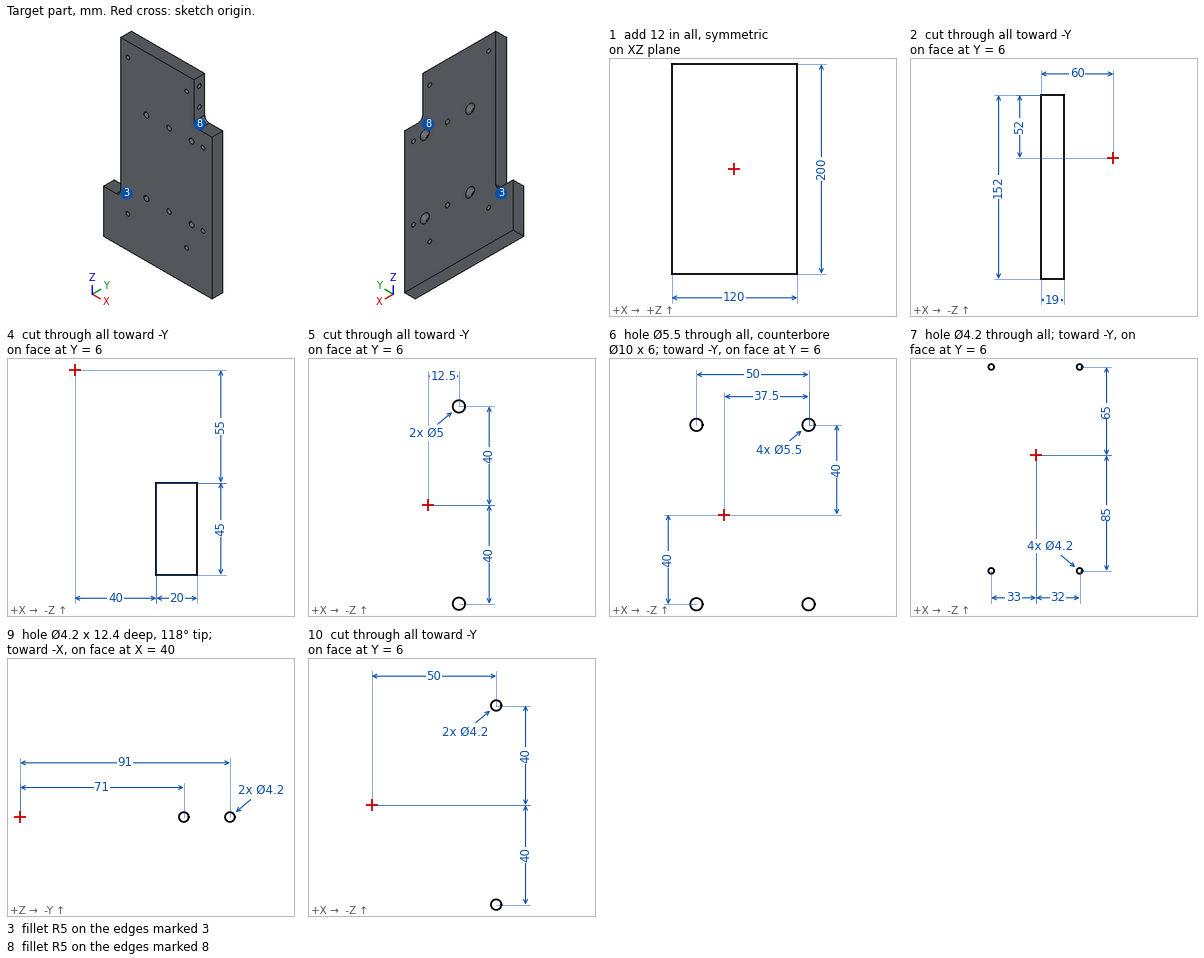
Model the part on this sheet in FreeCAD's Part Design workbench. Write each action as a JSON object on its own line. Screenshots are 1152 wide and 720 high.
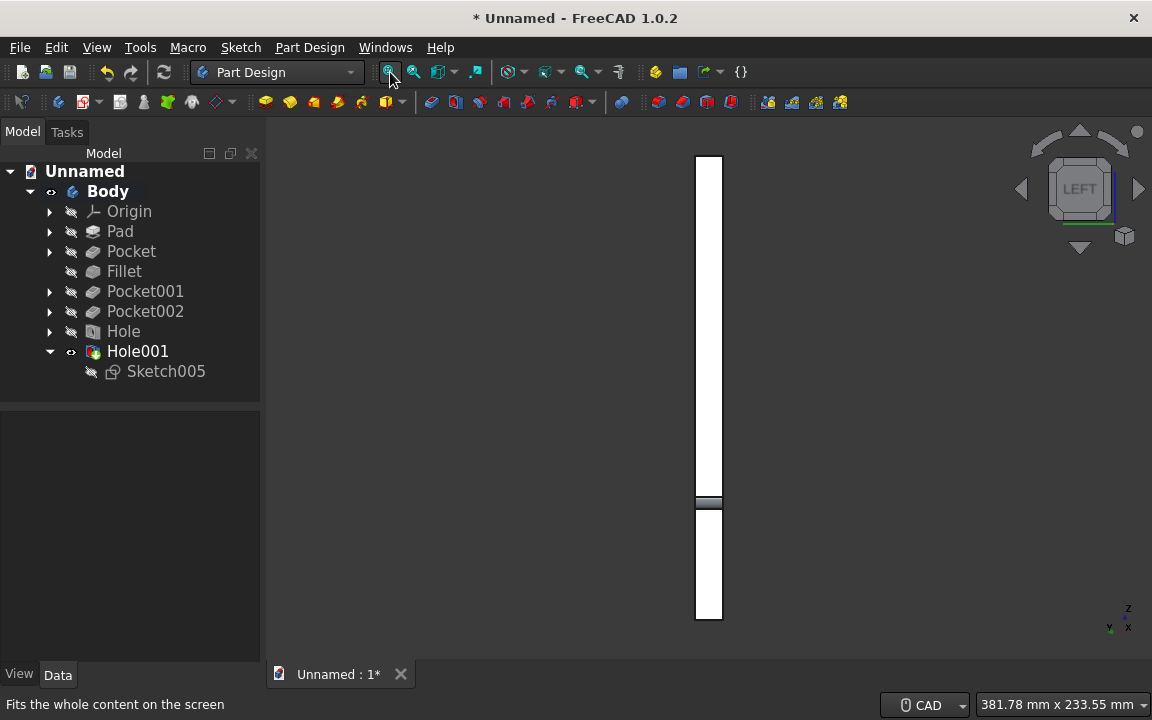
{"action": "key", "text": "v 3"}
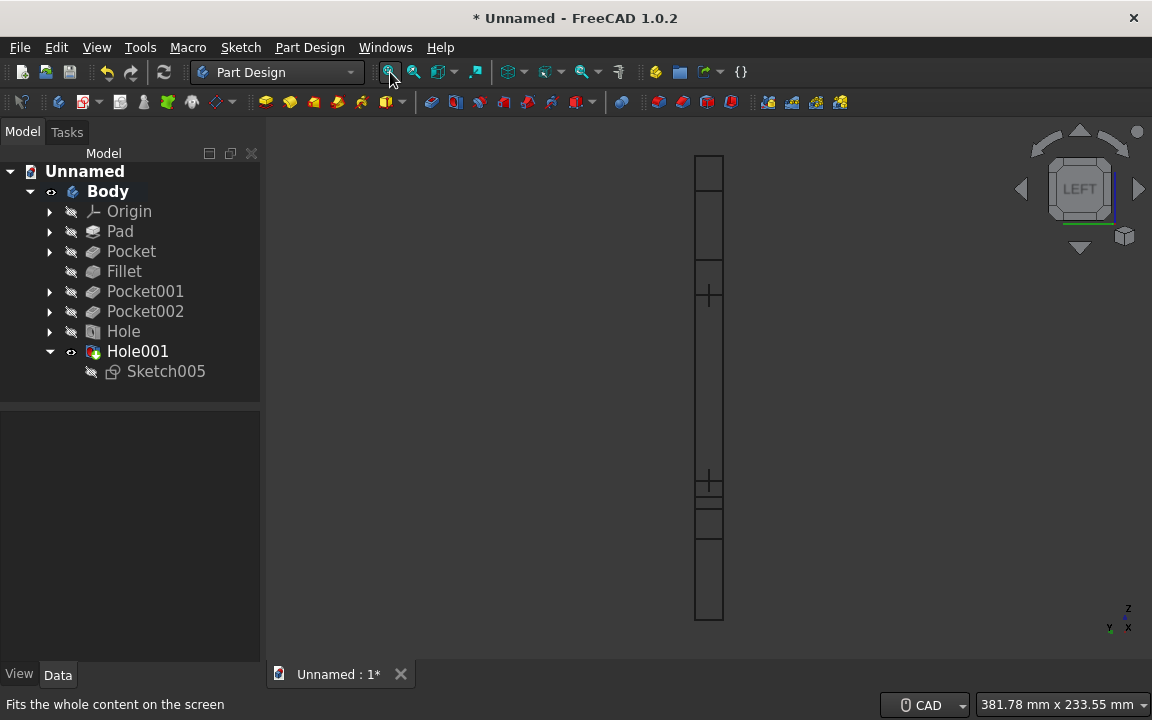
{"action": "key", "text": "0"}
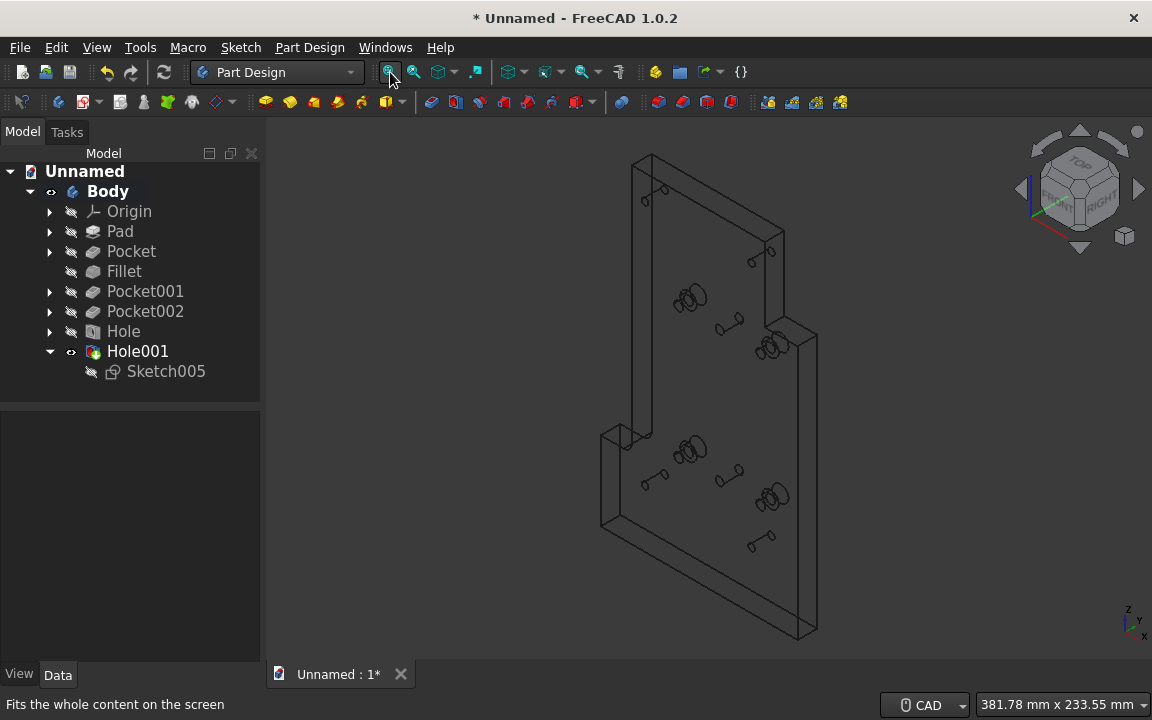
{"action": "left_click", "coordinate": [775, 321]}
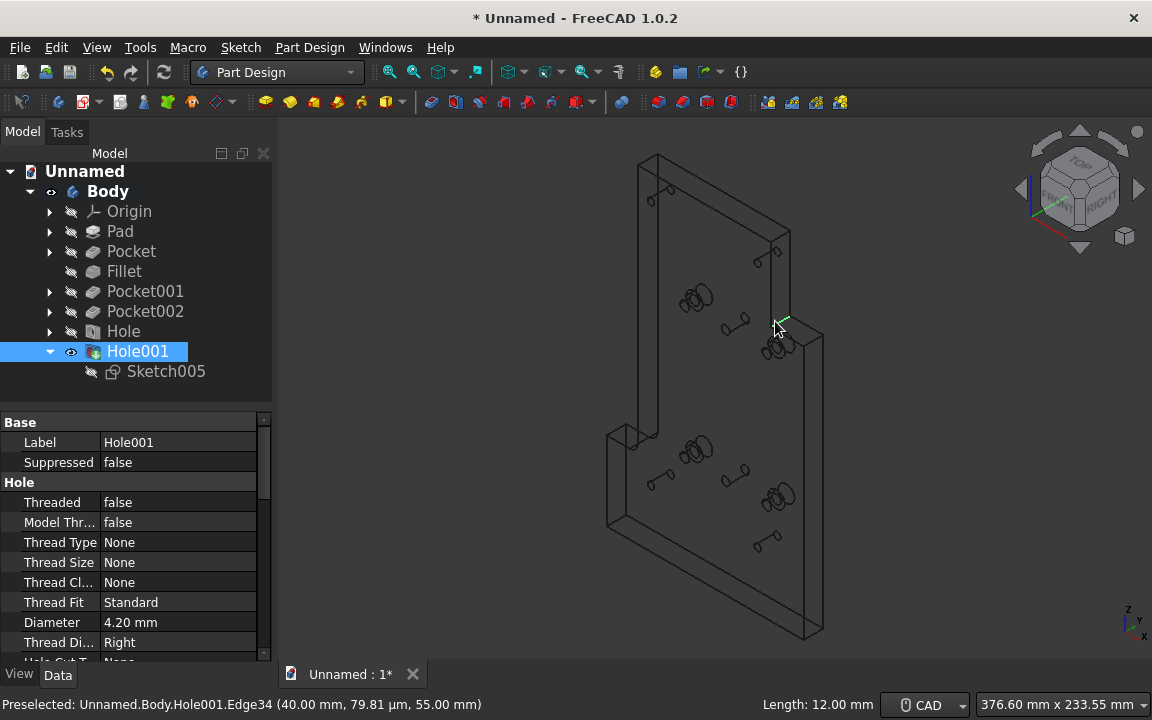
{"action": "key", "text": "v 1"}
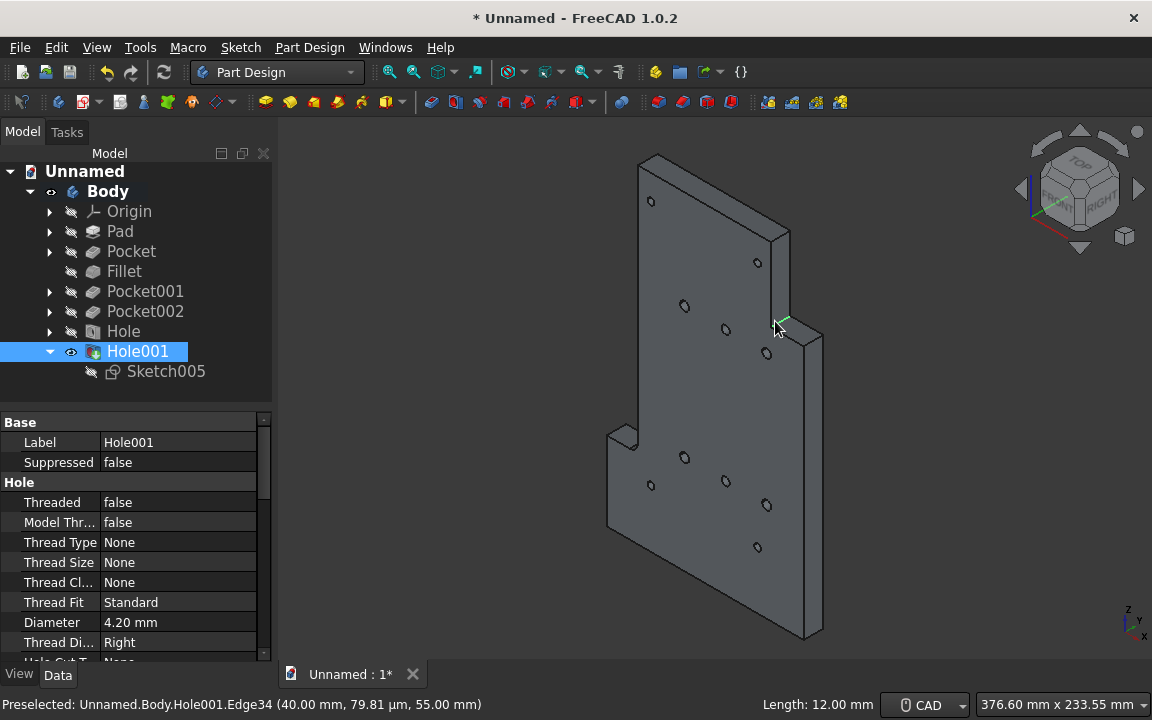
{"action": "left_click", "coordinate": [660, 102]}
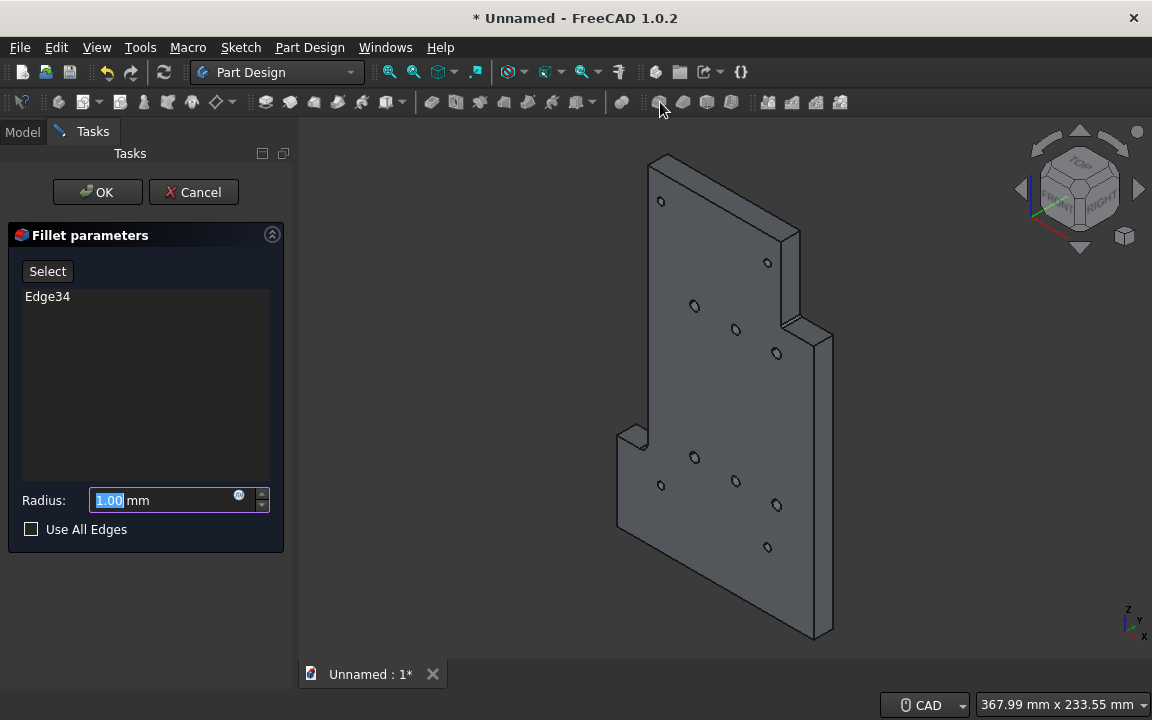
{"action": "type", "text": "5"}
{"action": "key", "text": "Tab"}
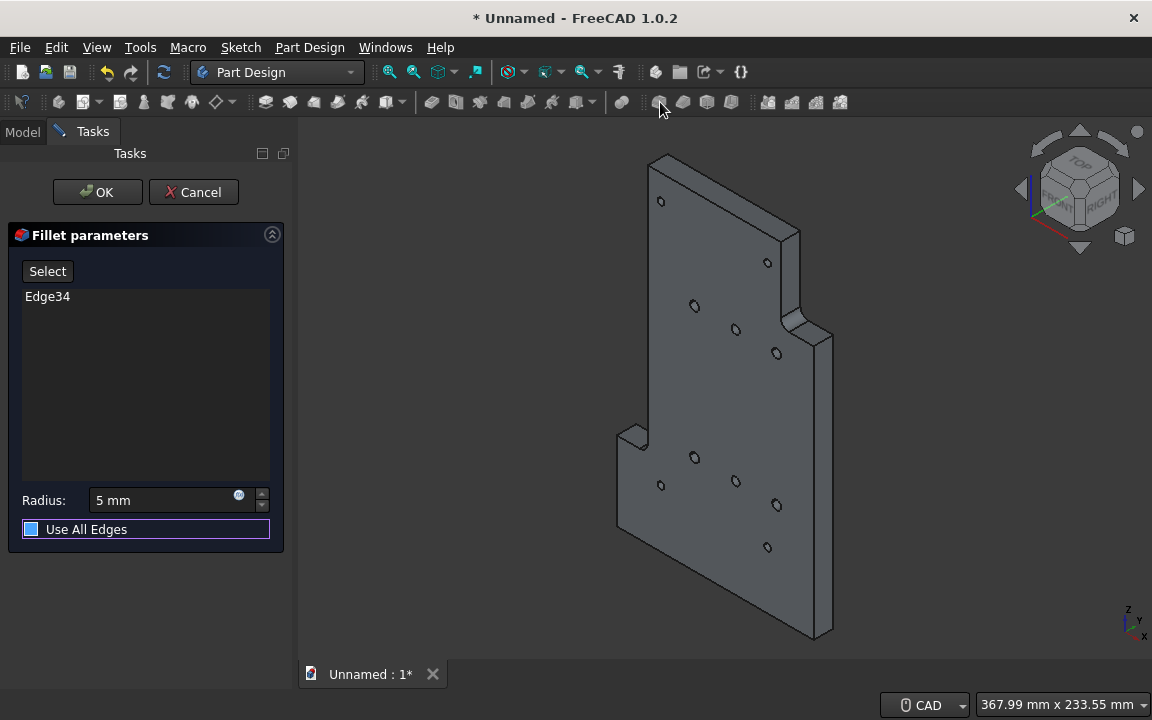
{"action": "left_click", "coordinate": [98, 192]}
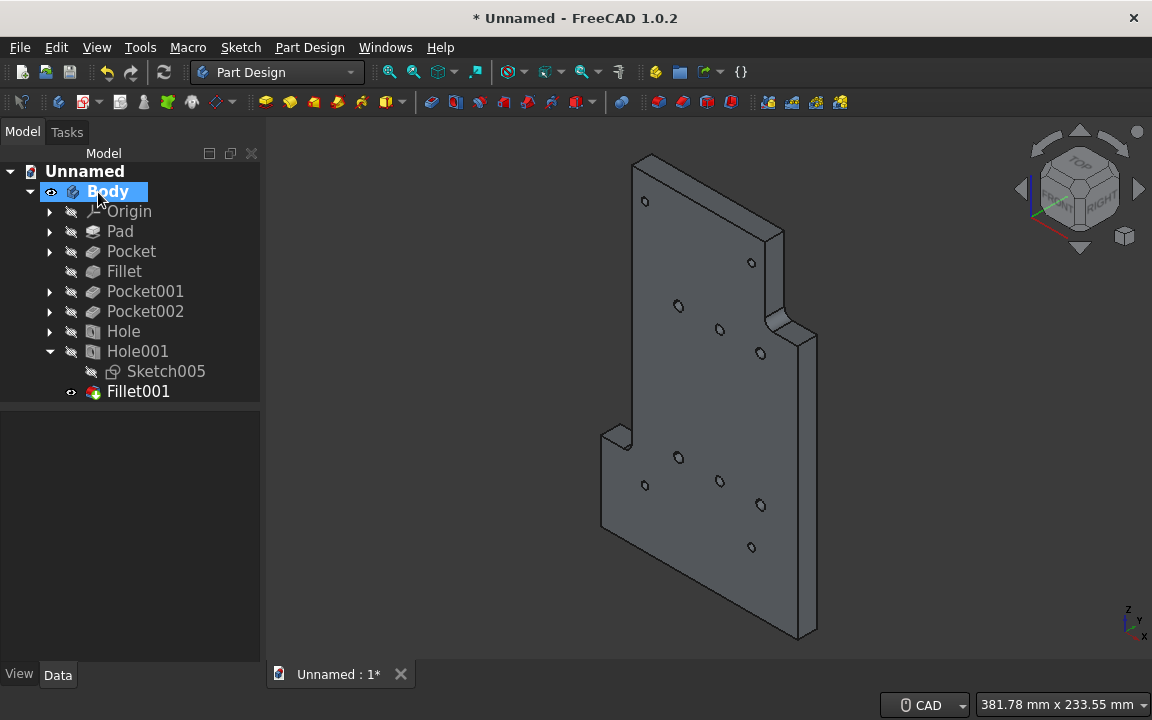
{"action": "left_click", "coordinate": [775, 295]}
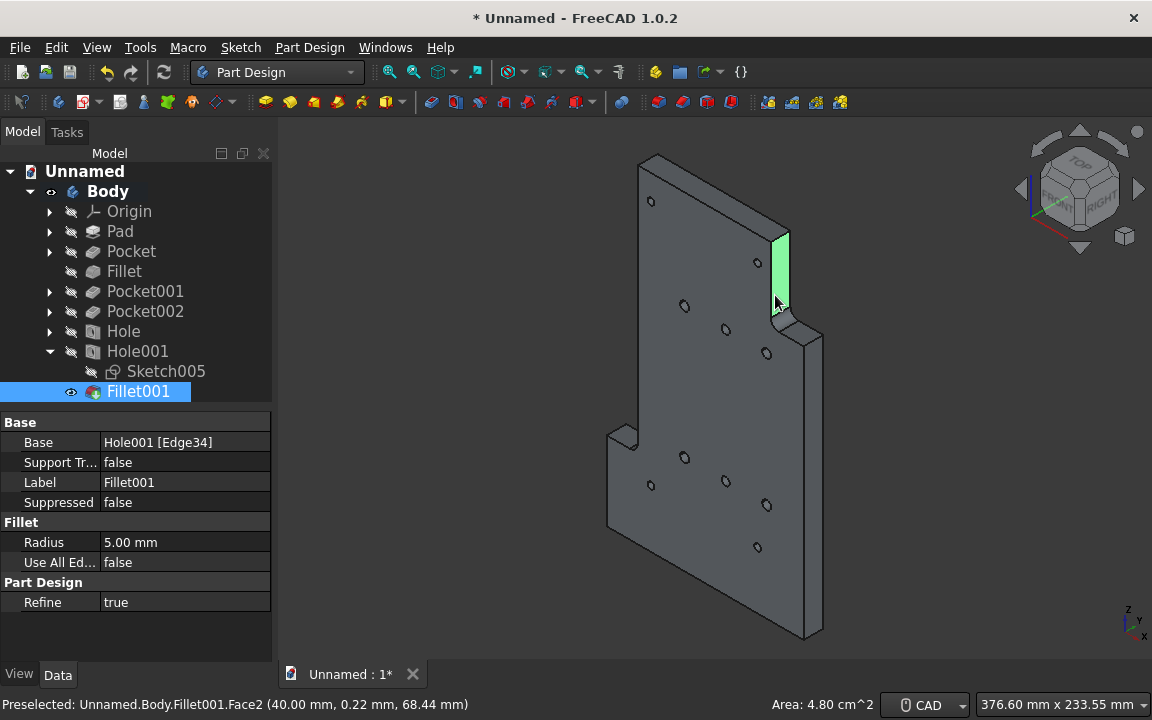
{"action": "left_click", "coordinate": [84, 102]}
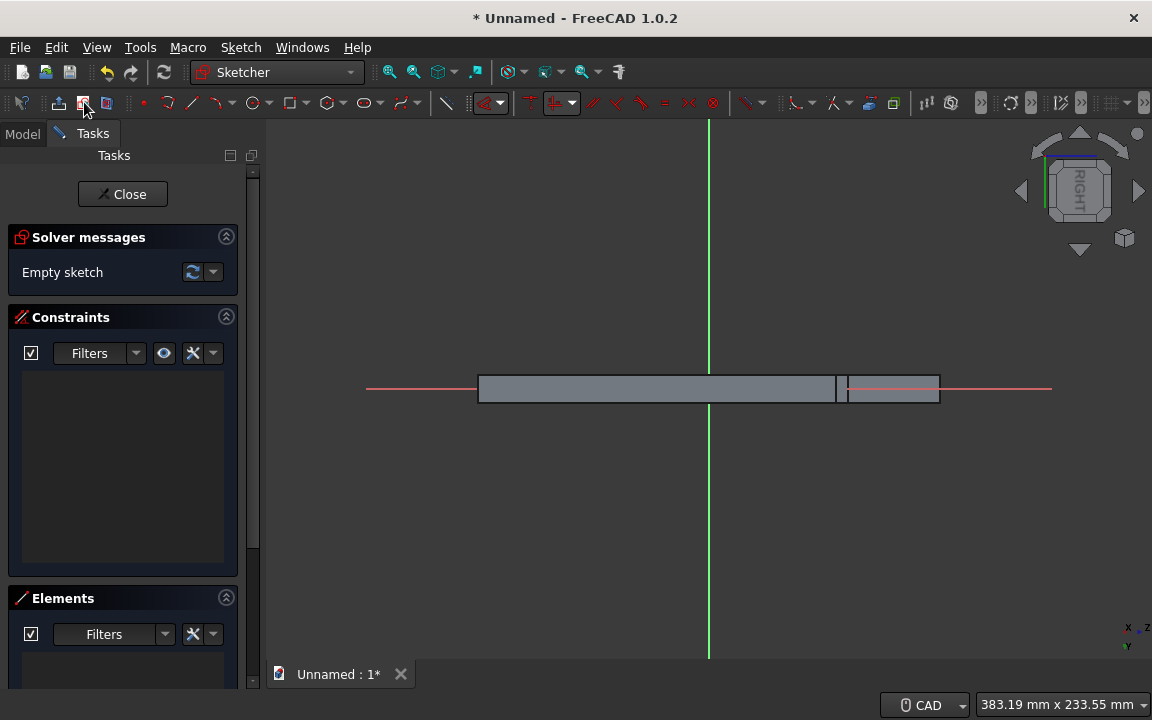
{"action": "left_click", "coordinate": [108, 104]}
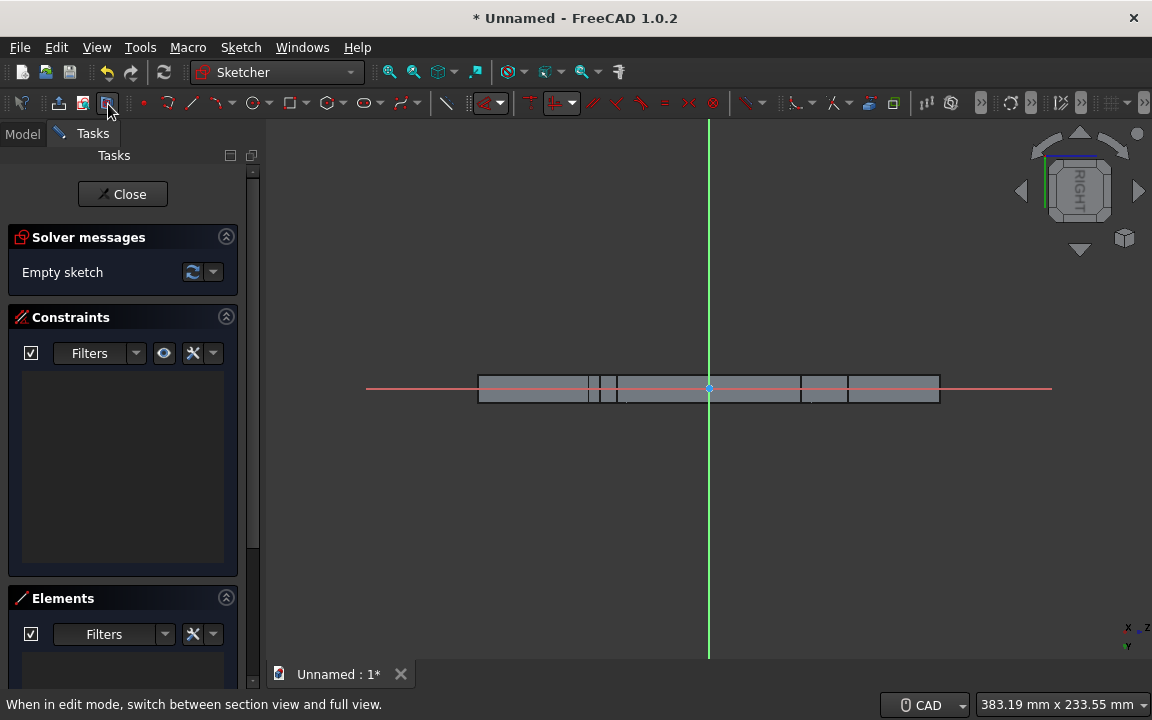
{"action": "scroll", "coordinate": [928, 389], "scroll_direction": "up", "scroll_amount": 11}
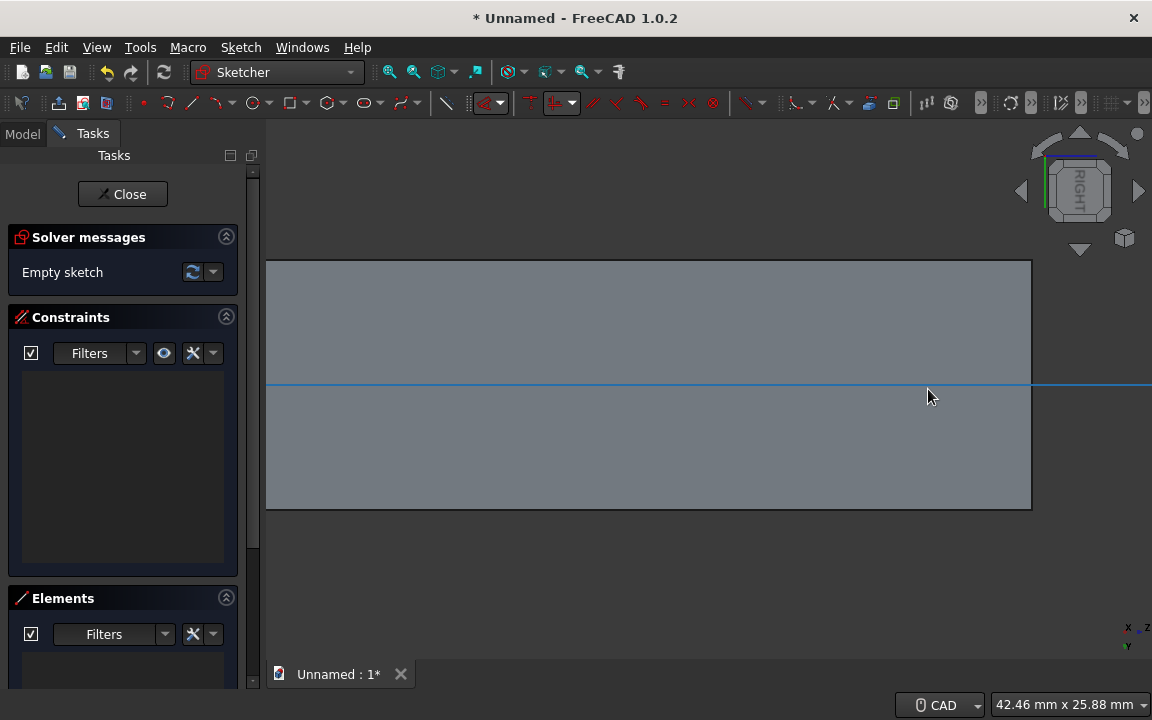
{"action": "left_click", "coordinate": [254, 104]}